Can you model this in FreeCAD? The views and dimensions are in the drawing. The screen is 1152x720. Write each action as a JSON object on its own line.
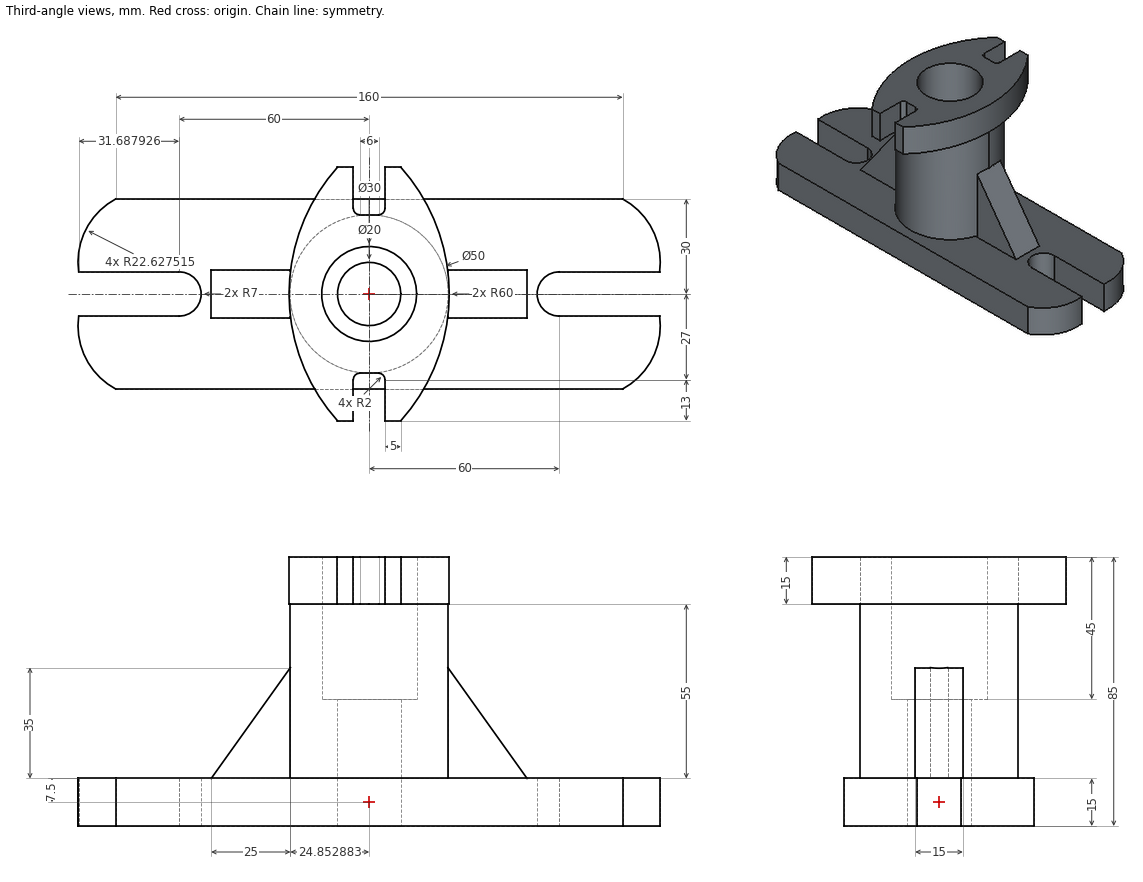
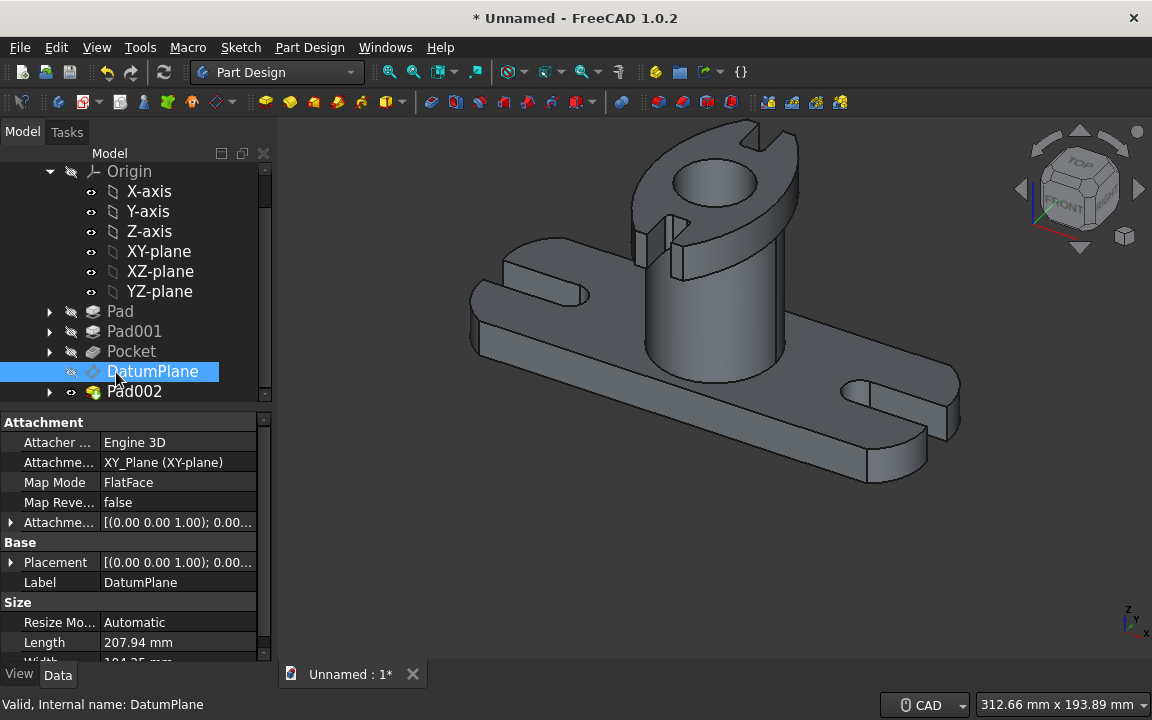
{"action": "key", "text": "v f"}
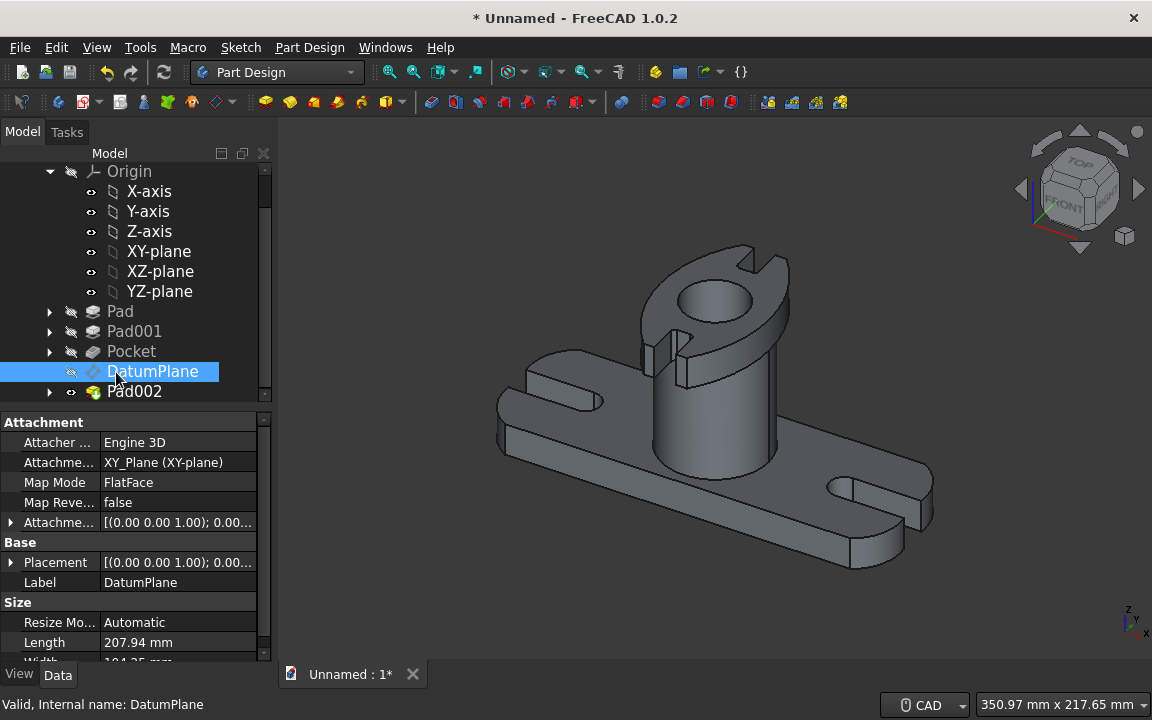
{"action": "left_click", "coordinate": [318, 619]}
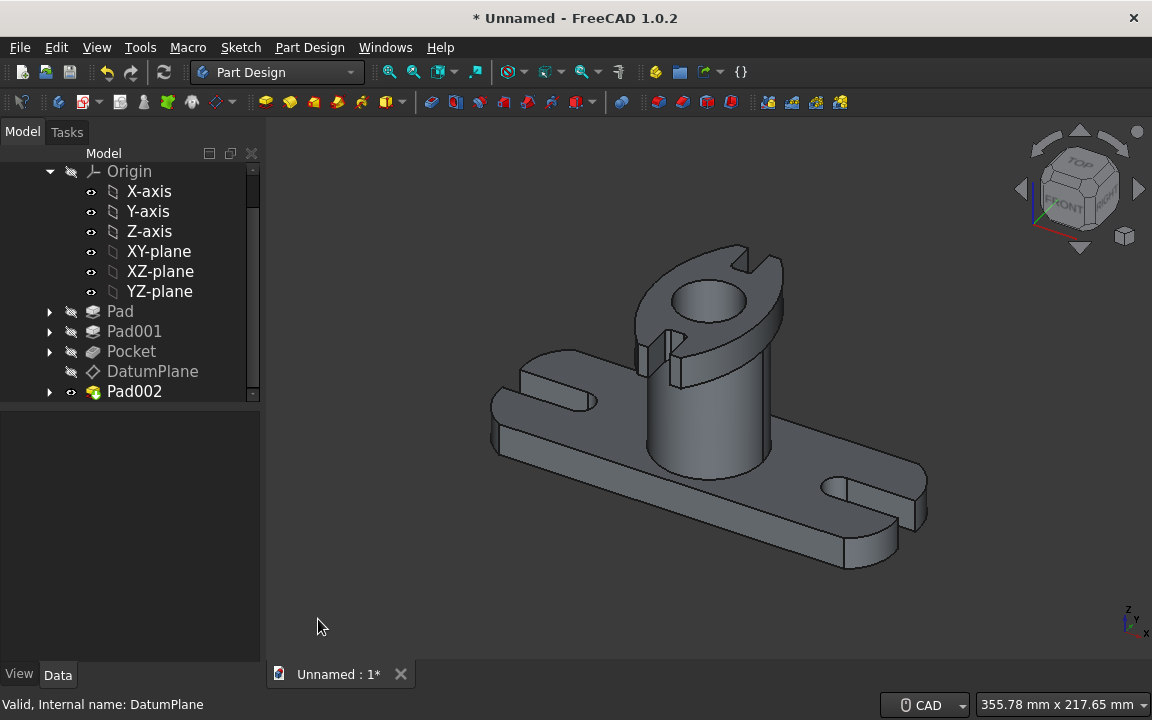
{"action": "left_click", "coordinate": [84, 102]}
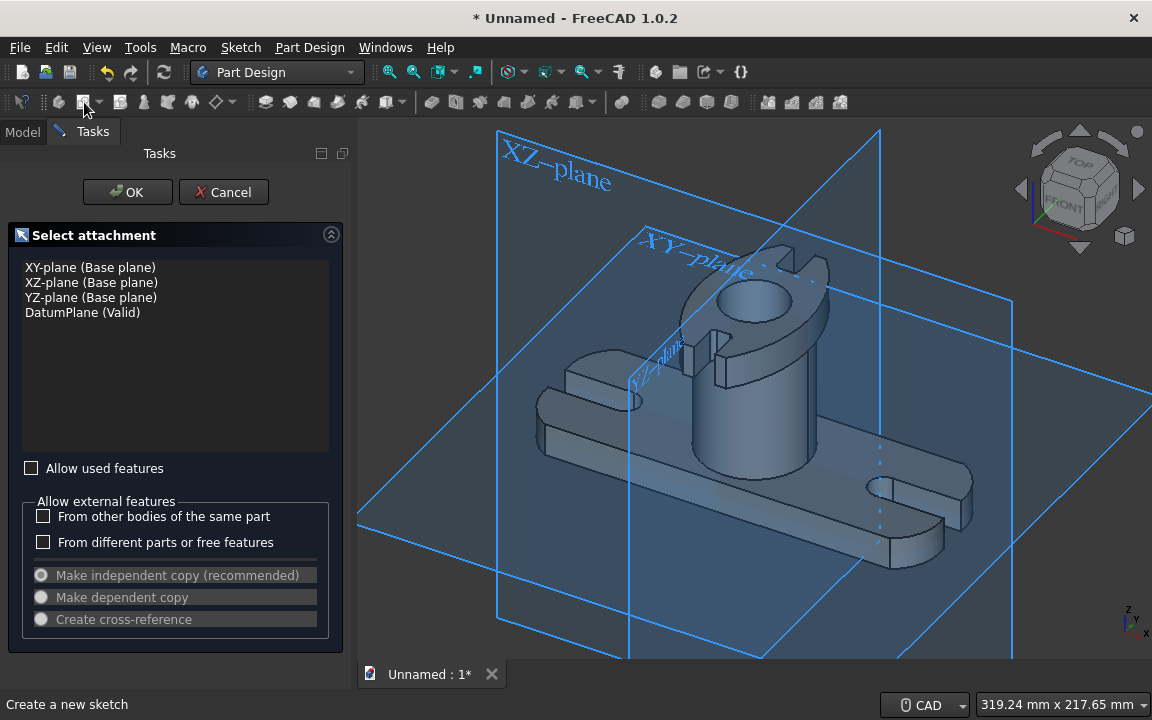
{"action": "left_click", "coordinate": [82, 282]}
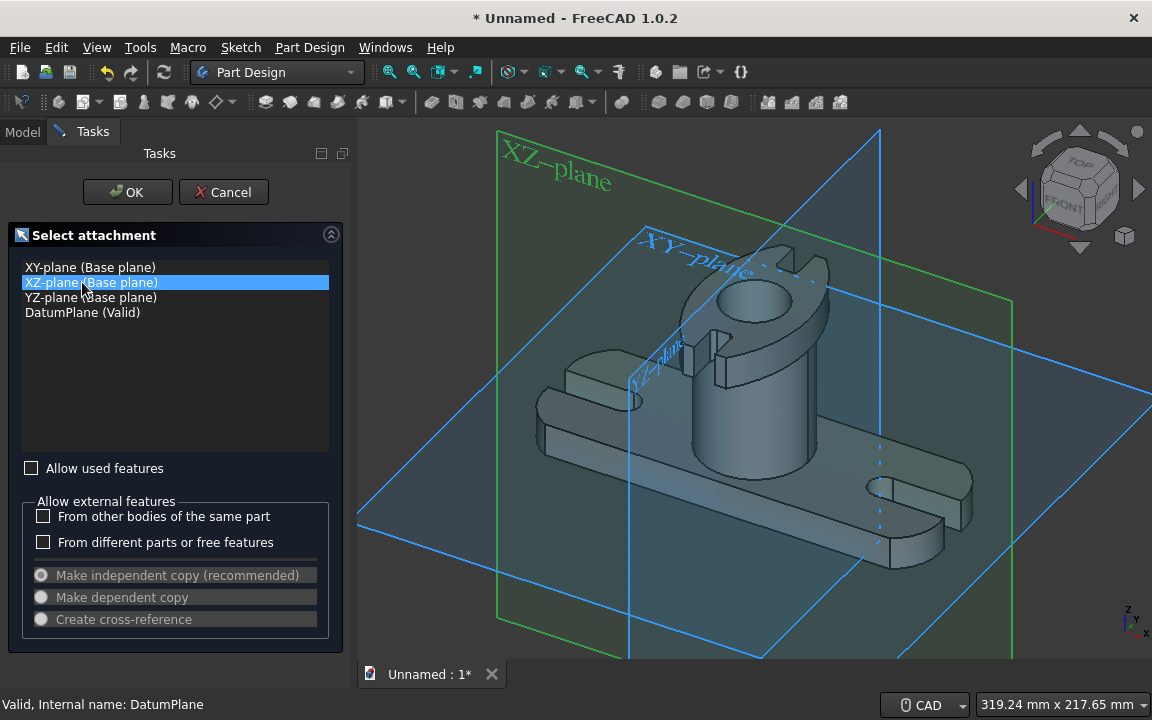
{"action": "left_click", "coordinate": [128, 192]}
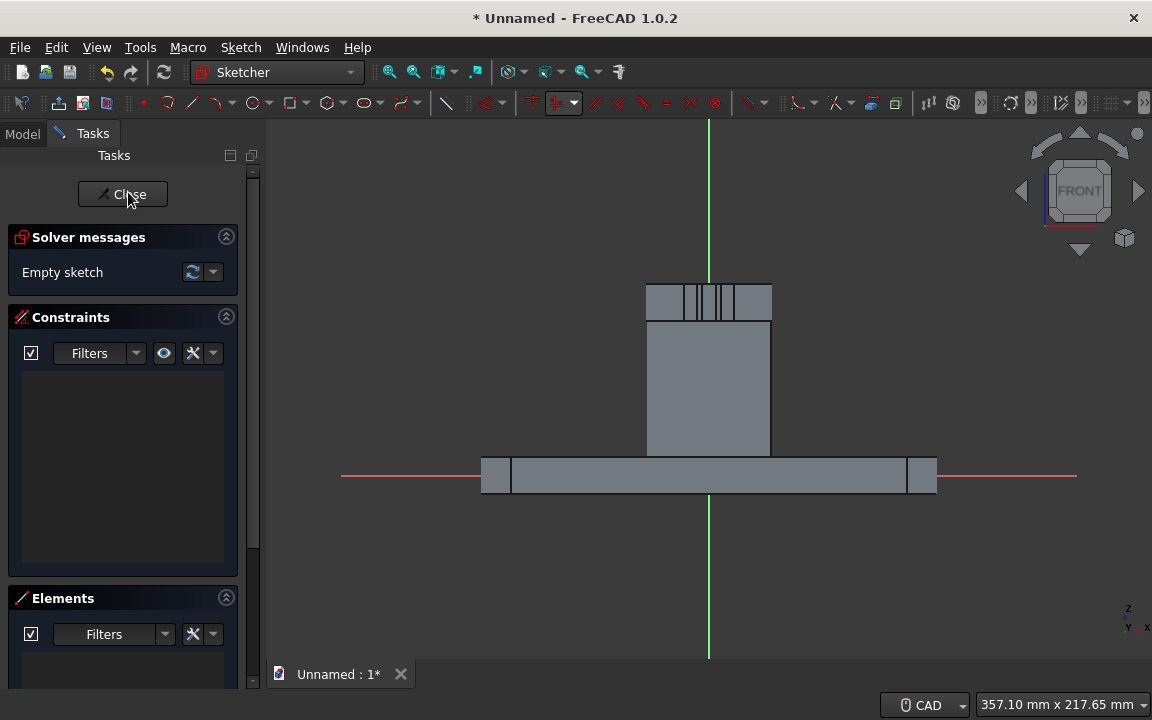
{"action": "key", "text": "q s"}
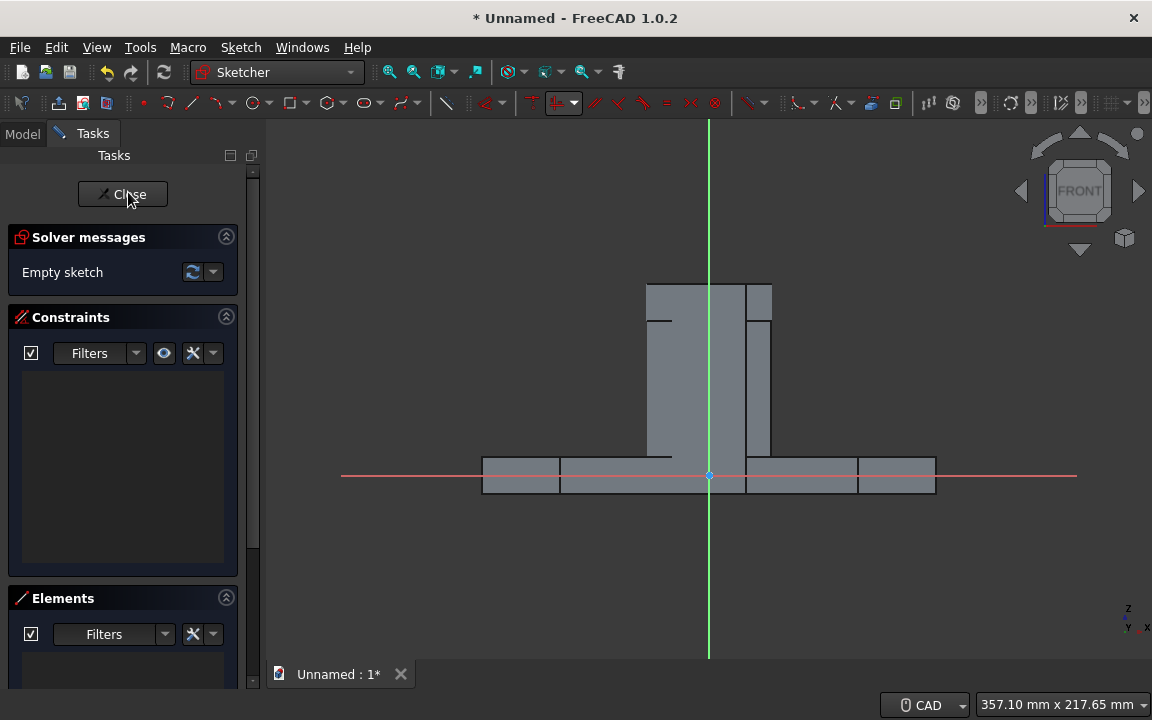
{"action": "scroll", "coordinate": [650, 438], "scroll_direction": "up", "scroll_amount": 6}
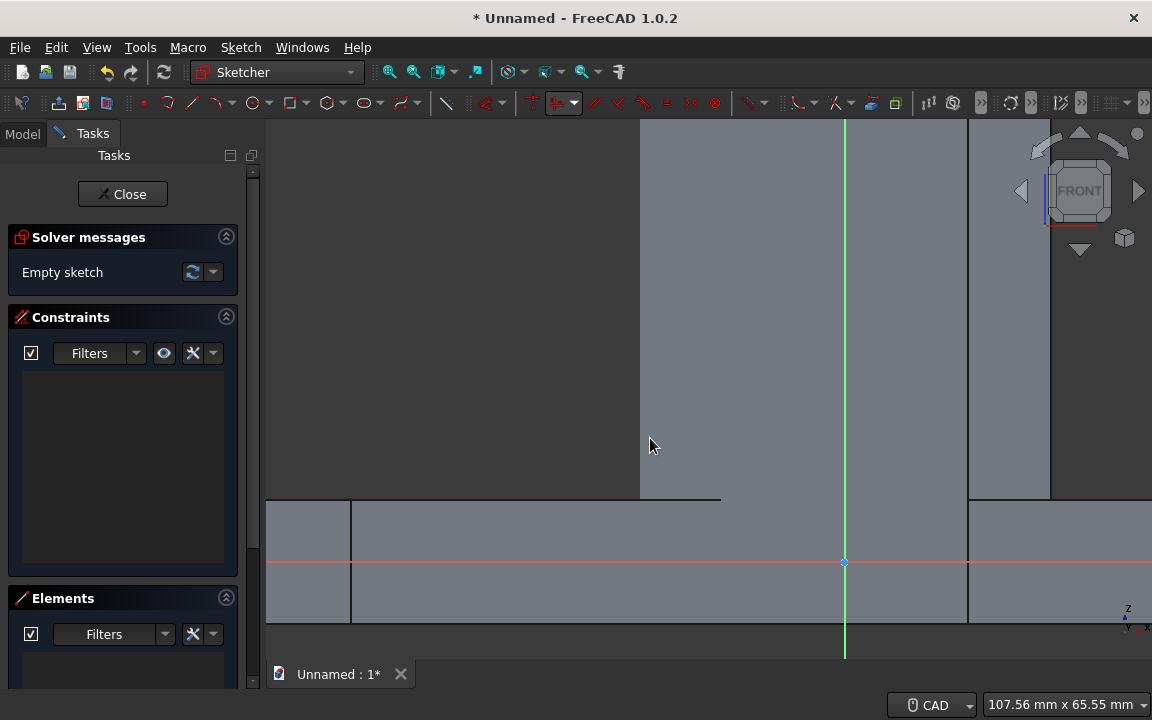
{"action": "key", "text": "g m"}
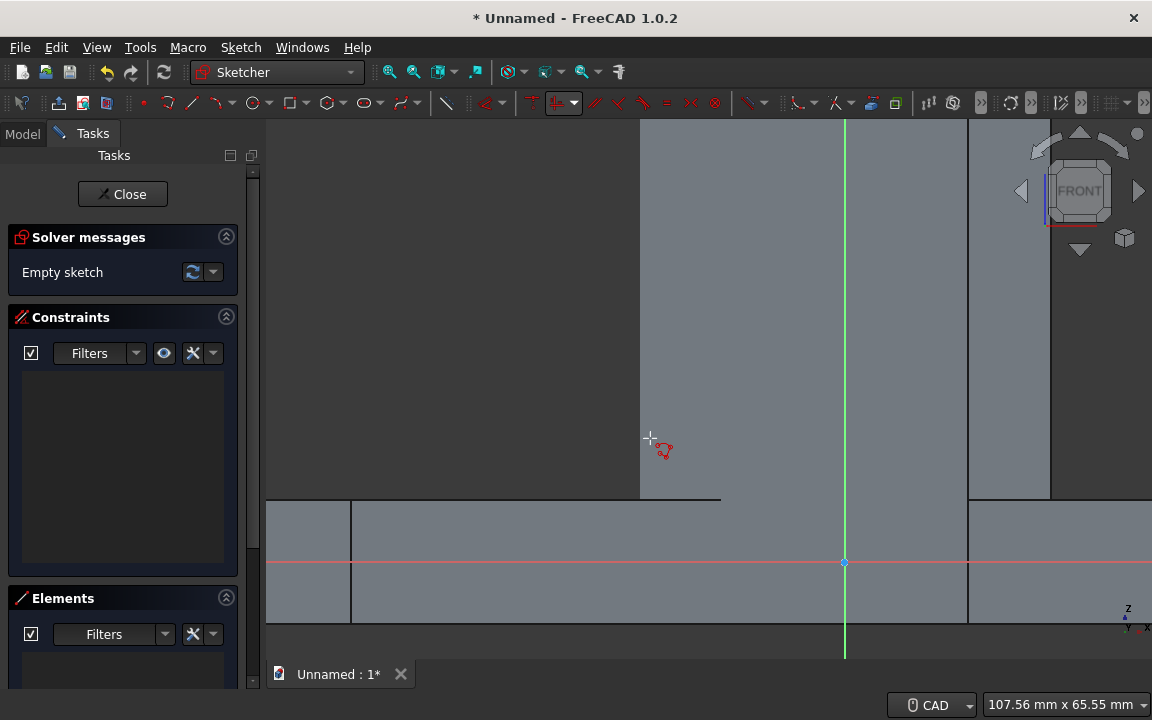
{"action": "left_click", "coordinate": [640, 500]}
{"action": "left_click", "coordinate": [434, 500]}
{"action": "left_click", "coordinate": [640, 212]}
{"action": "left_click", "coordinate": [640, 501]}
{"action": "key", "text": "Escape"}
{"action": "key", "text": "Escape"}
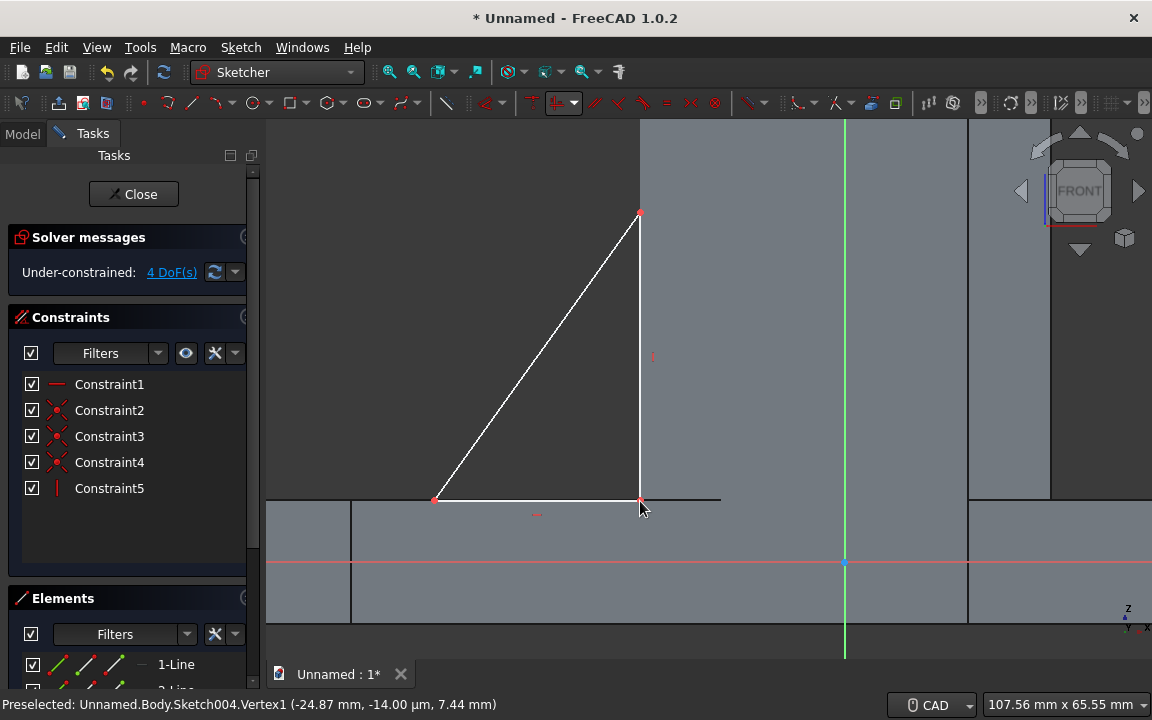
{"action": "key", "text": "d"}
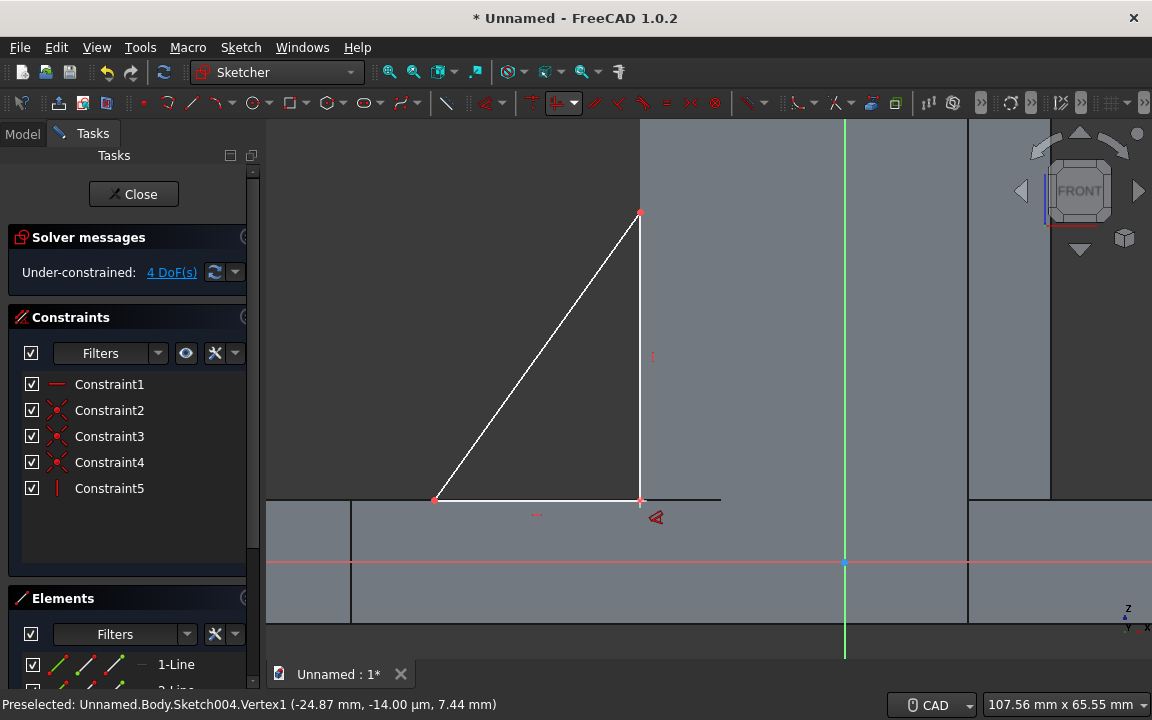
{"action": "left_click", "coordinate": [578, 501]}
{"action": "left_click", "coordinate": [537, 535]}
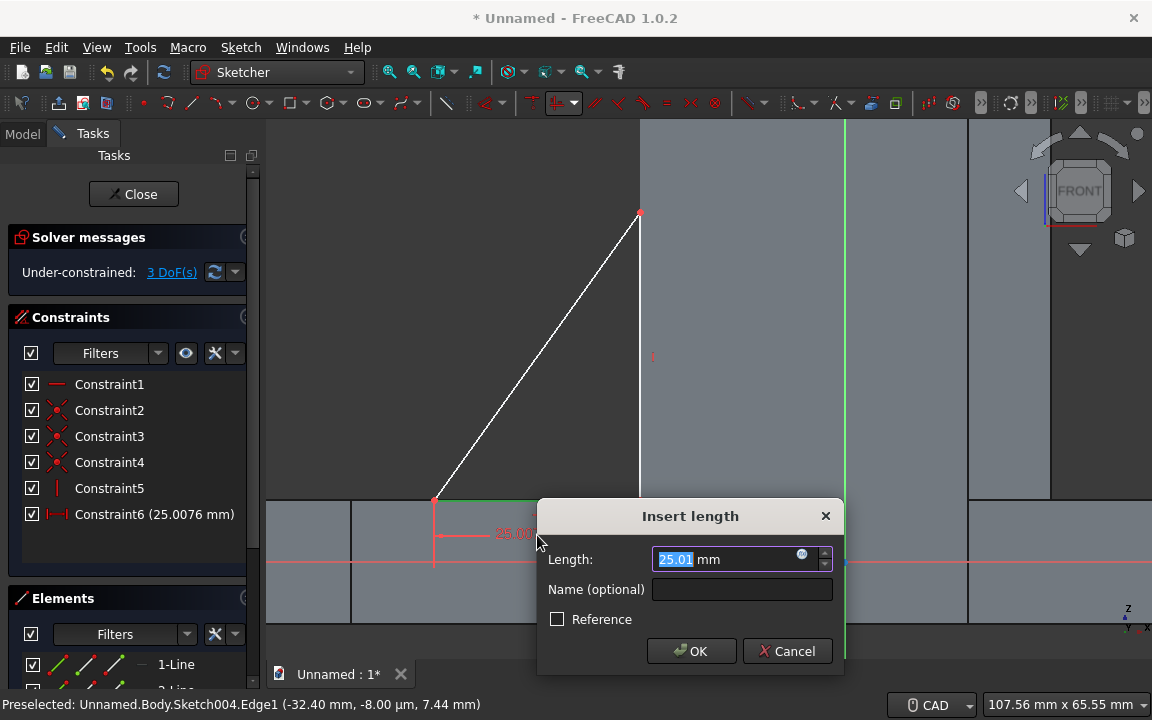
{"action": "type", "text": "25"}
{"action": "key", "text": "Return"}